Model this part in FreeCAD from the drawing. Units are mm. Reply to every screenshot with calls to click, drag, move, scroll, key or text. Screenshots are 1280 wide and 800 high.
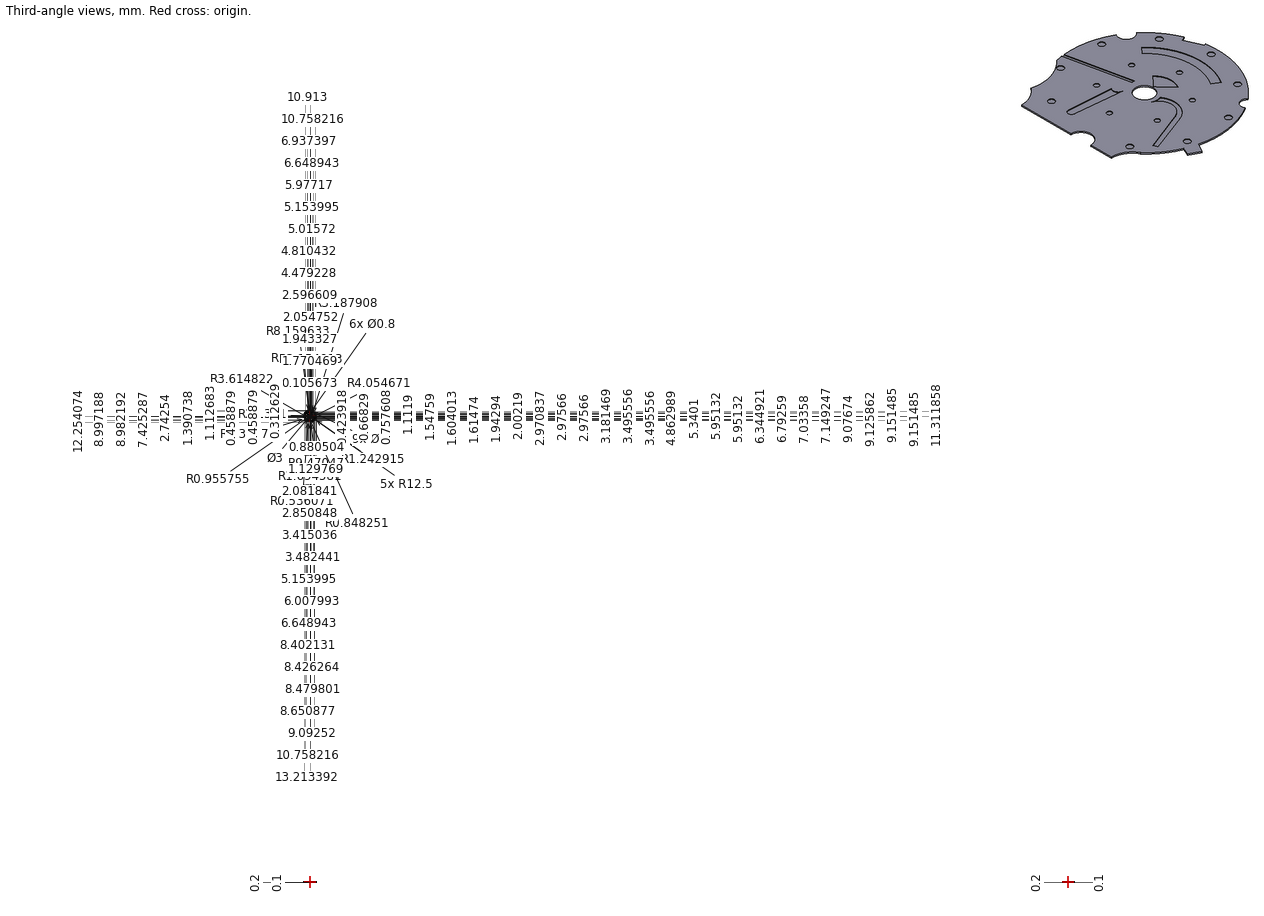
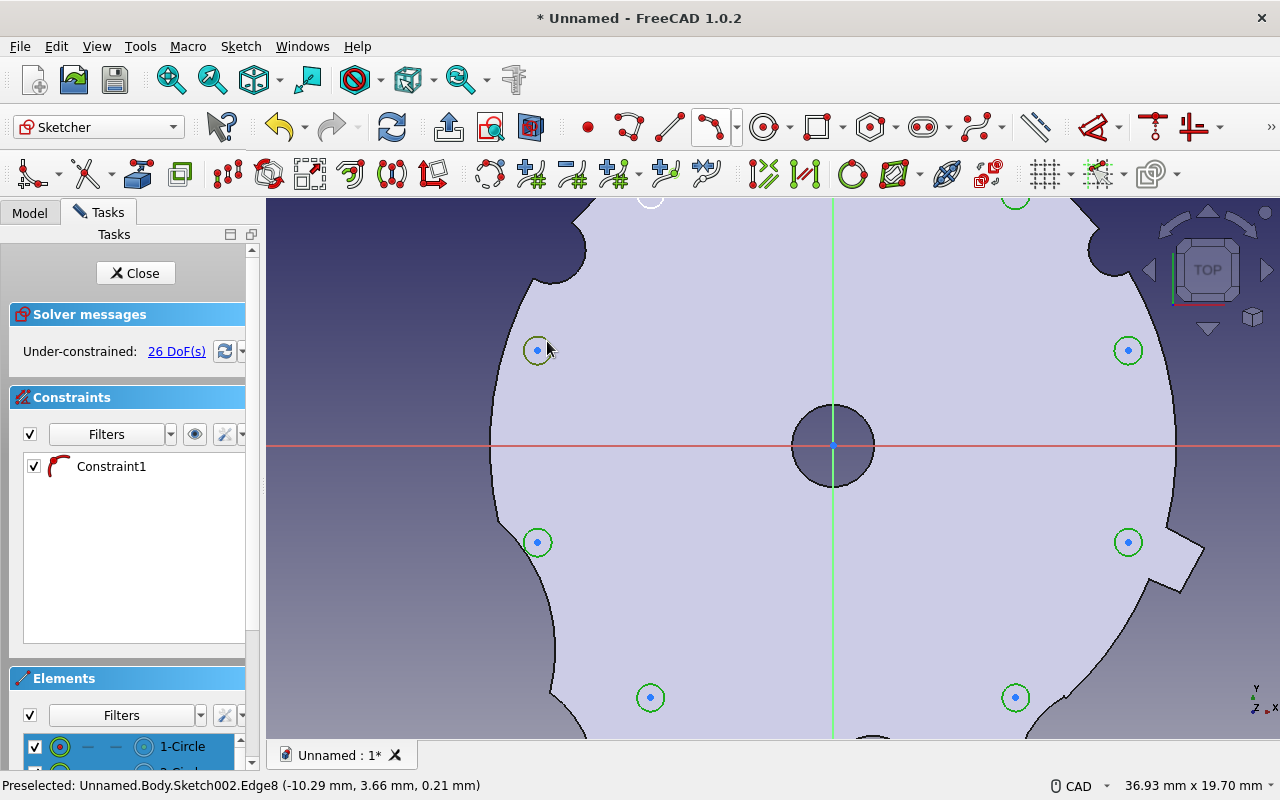
scroll(548, 532, down, 3)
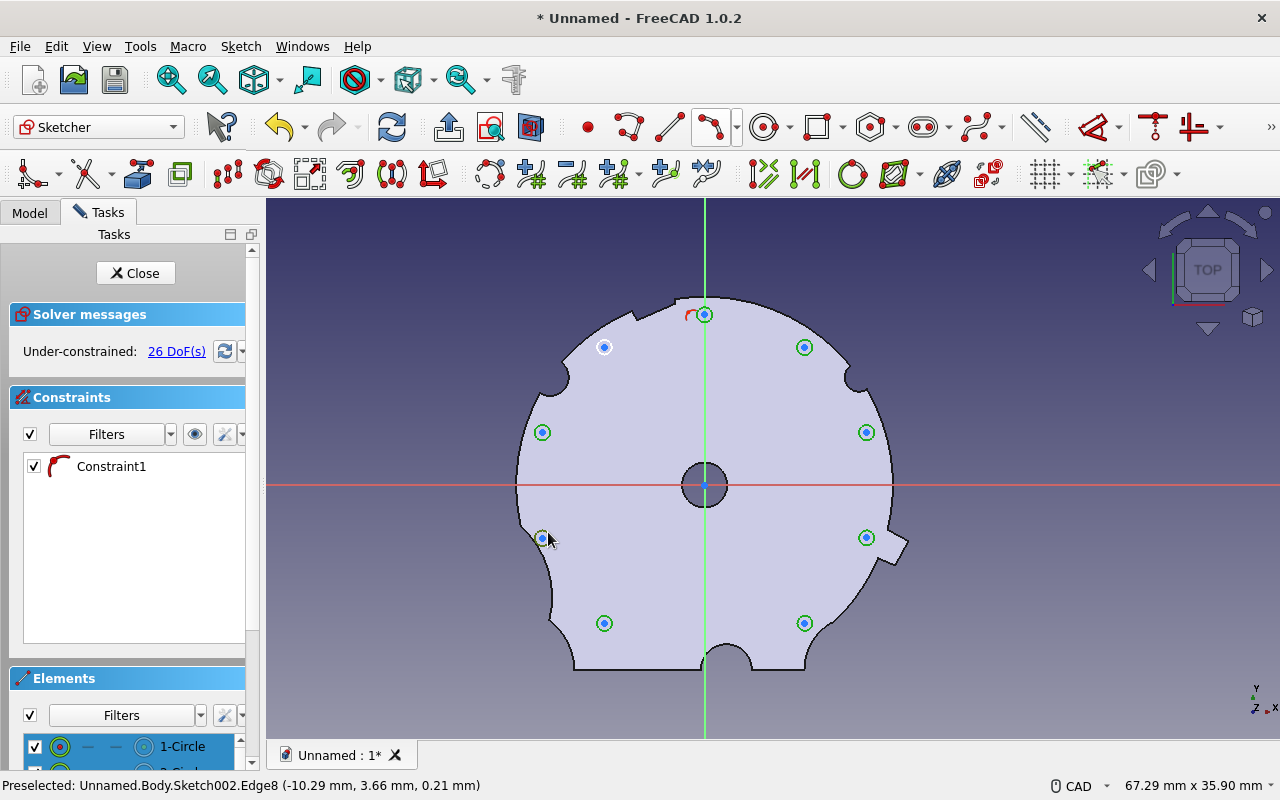
scroll(610, 342, up, 4)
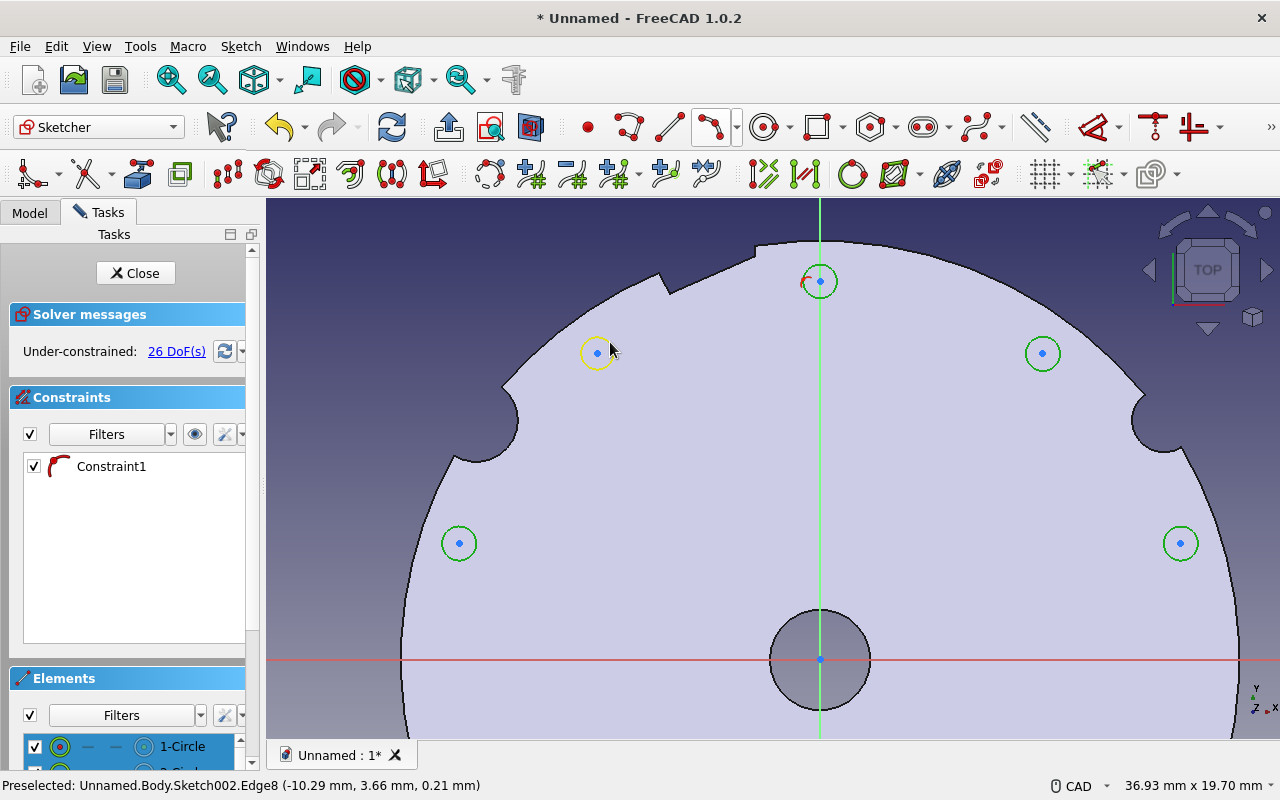
click(609, 342)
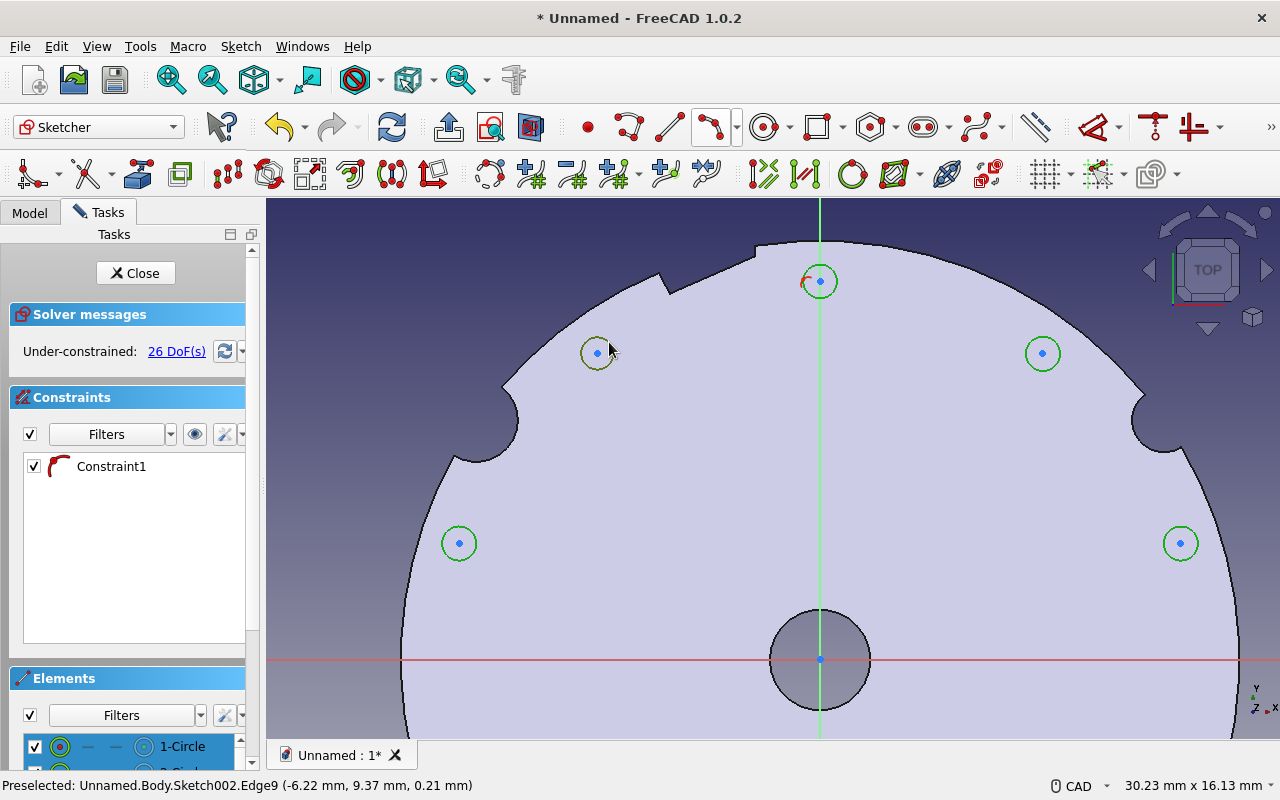
key(e)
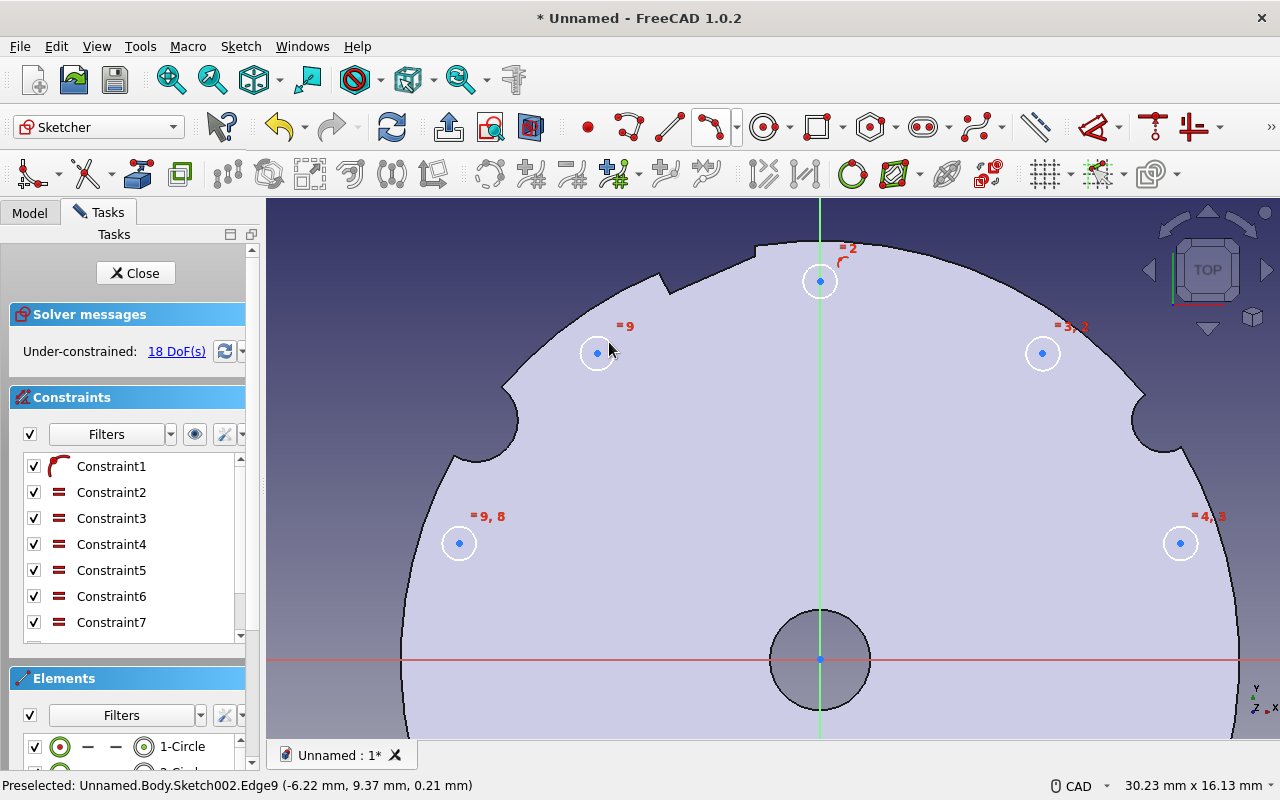
key(d)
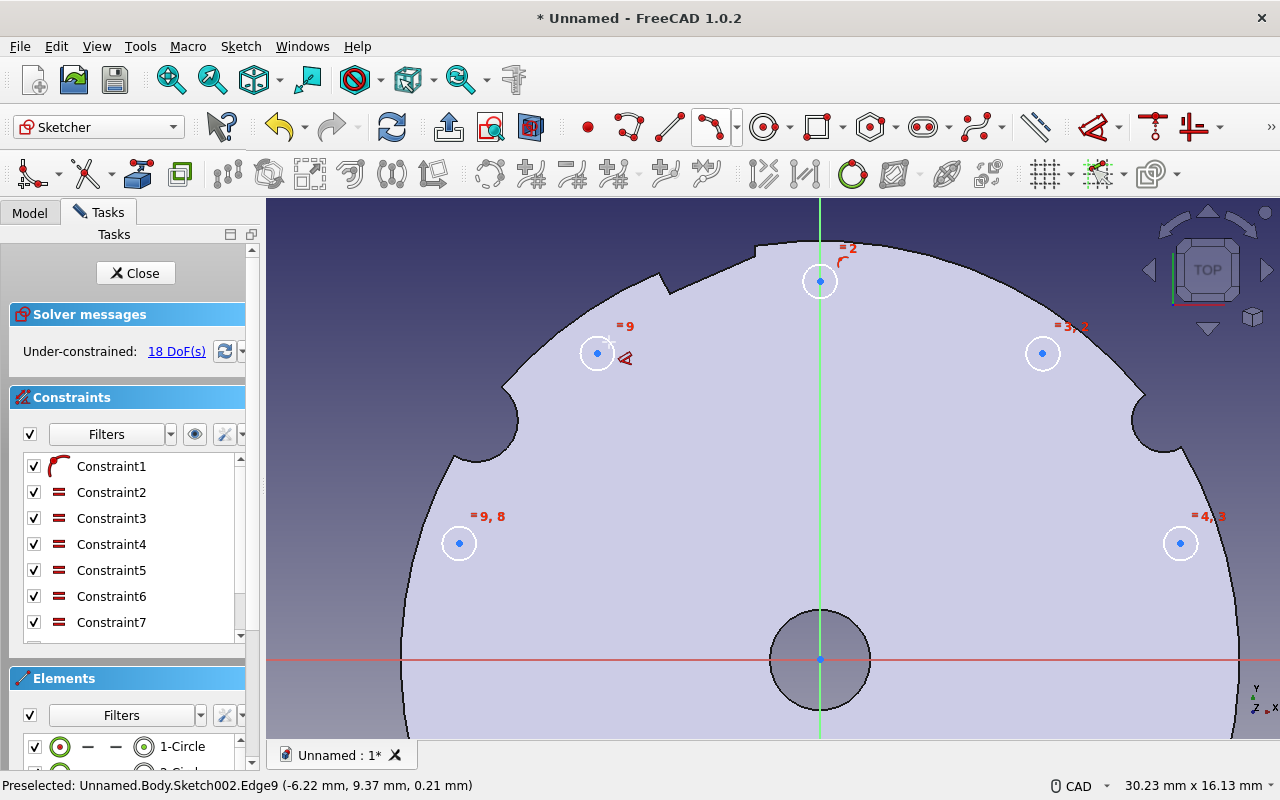
click(832, 270)
click(855, 248)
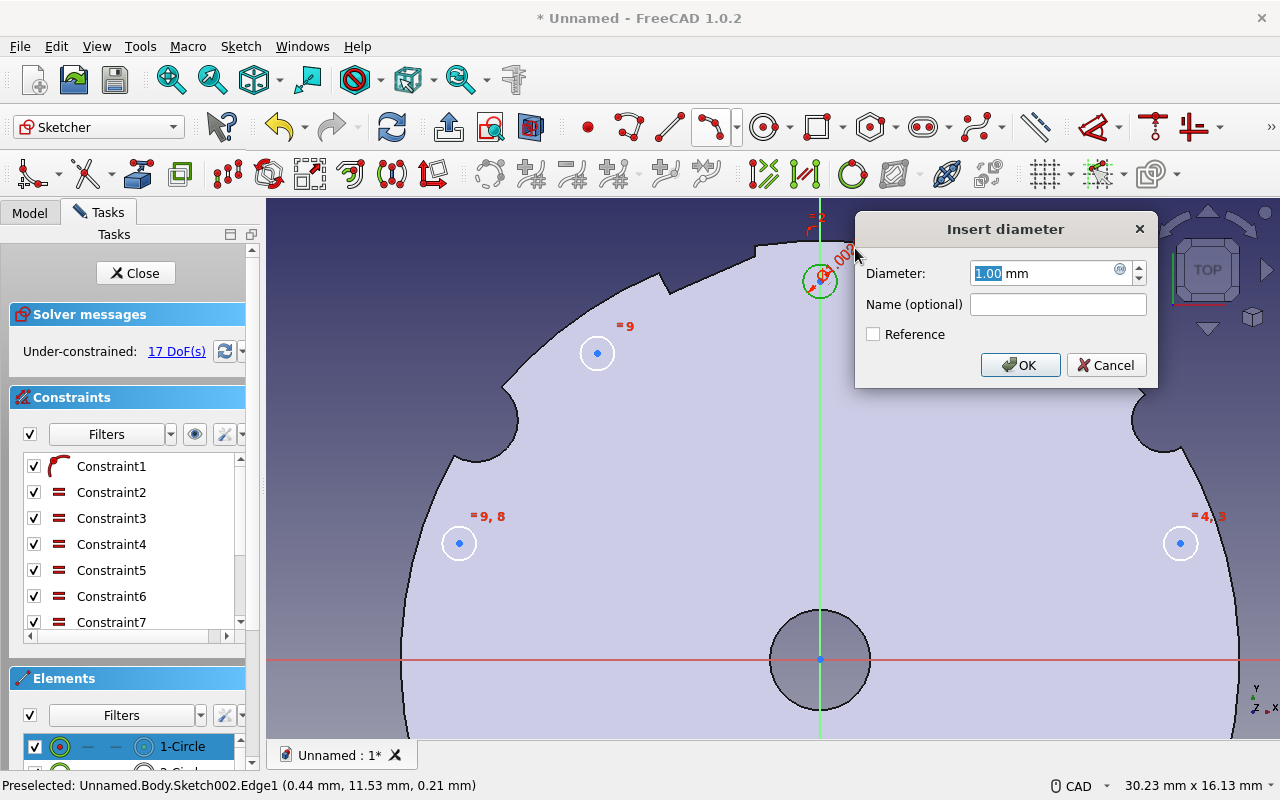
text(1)
key(Return)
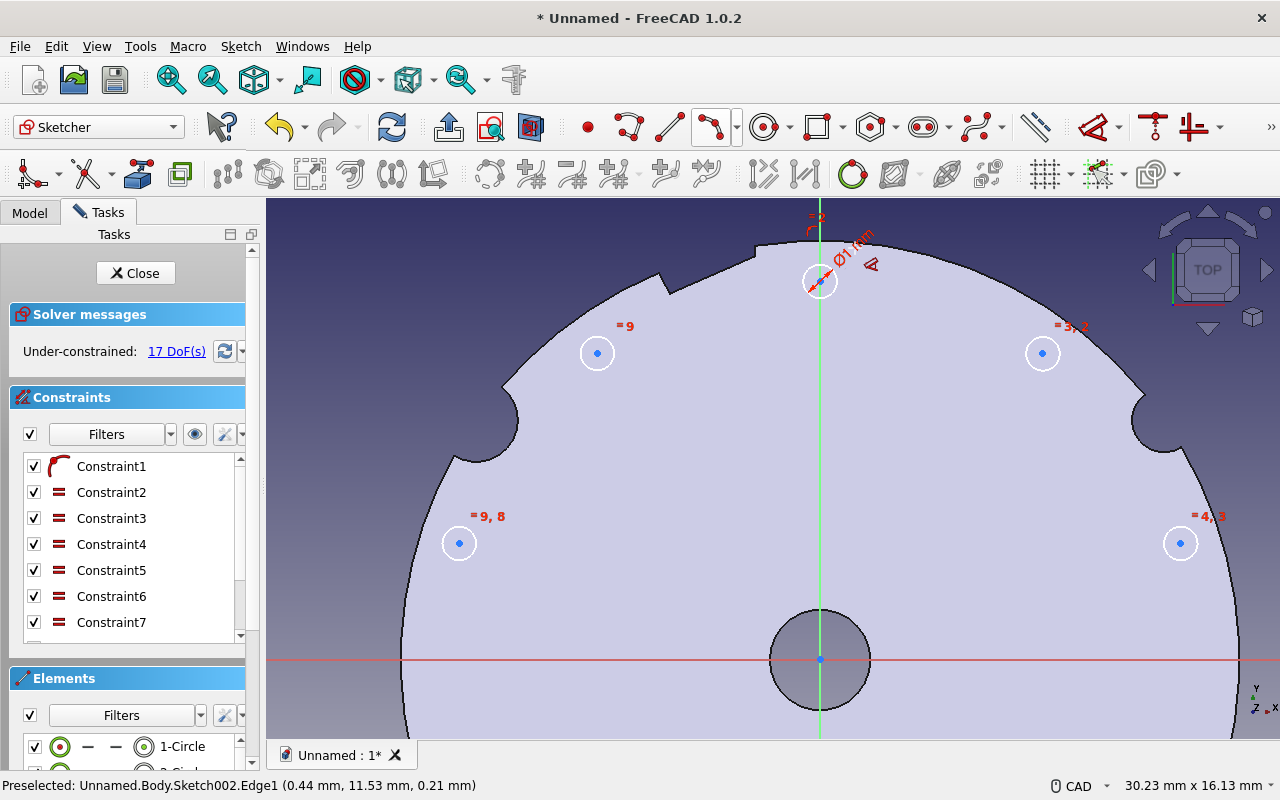
click(1043, 354)
click(932, 320)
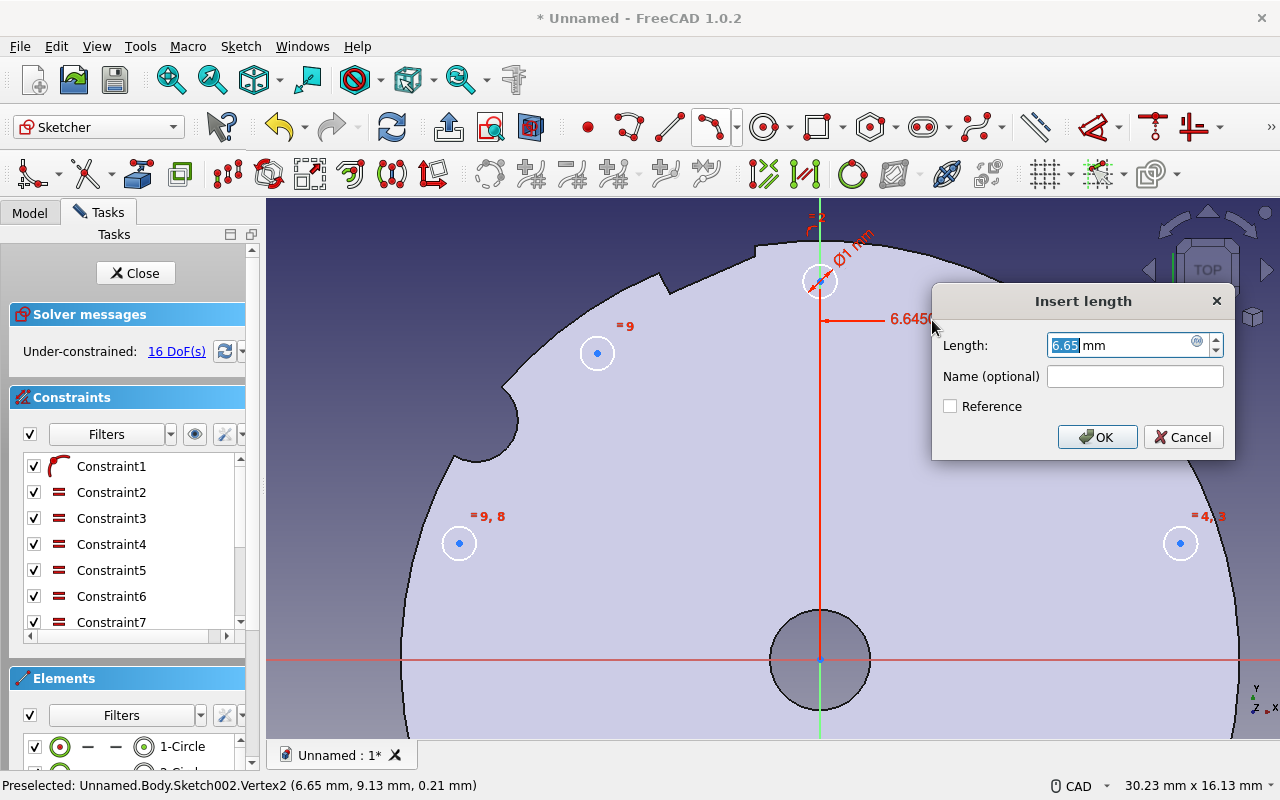
text(6.648943)
key(Return)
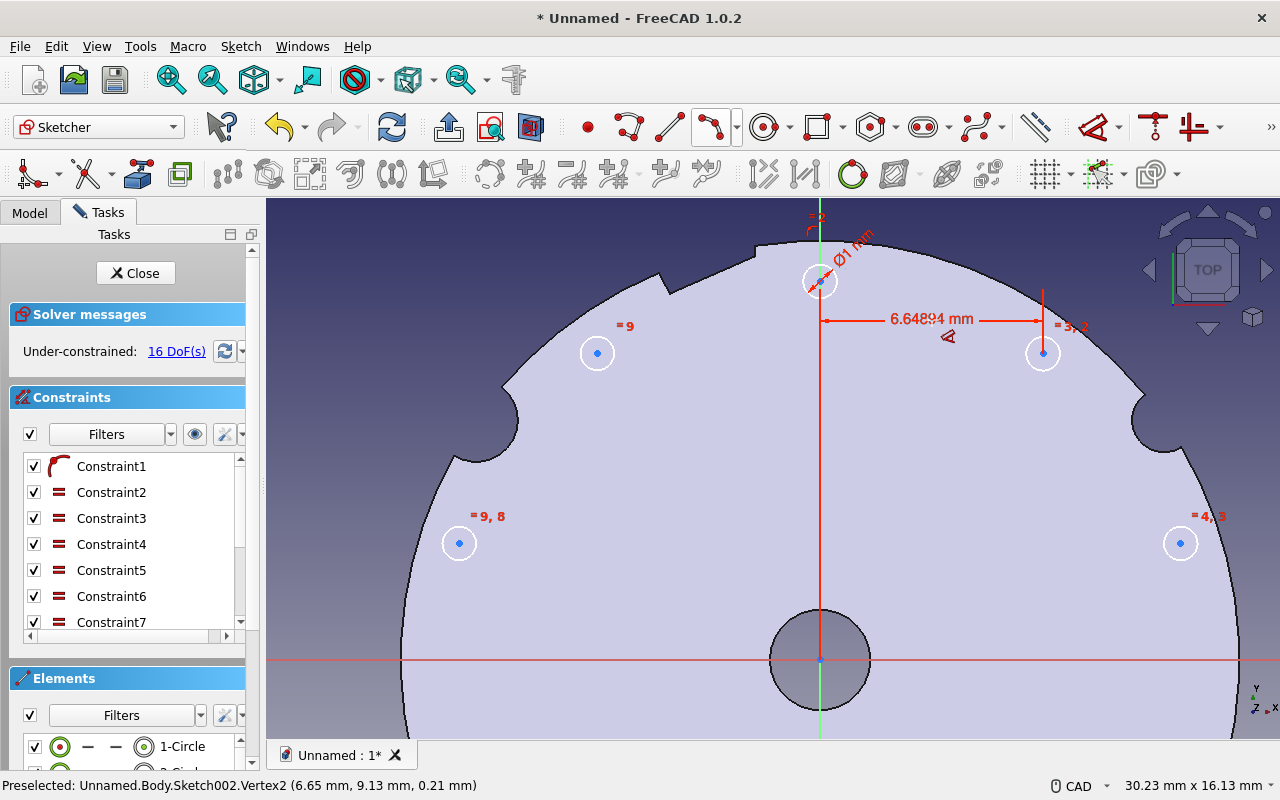
click(1043, 354)
click(1077, 507)